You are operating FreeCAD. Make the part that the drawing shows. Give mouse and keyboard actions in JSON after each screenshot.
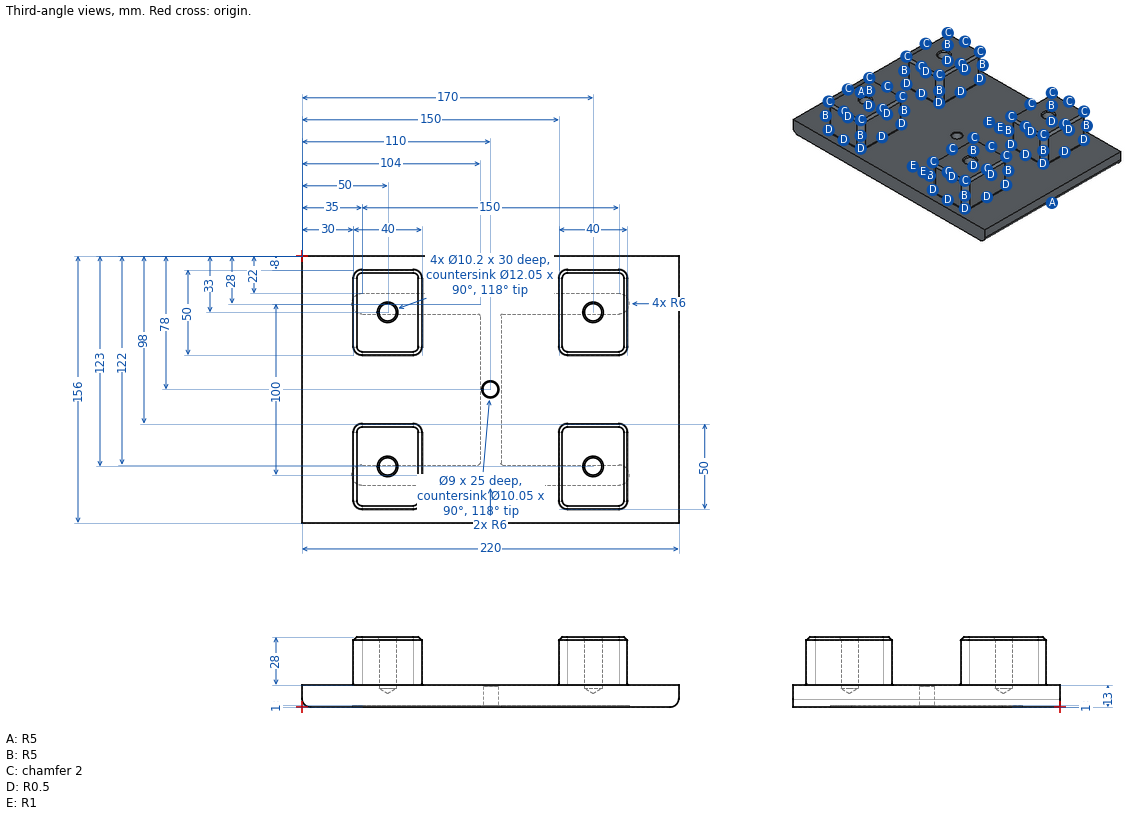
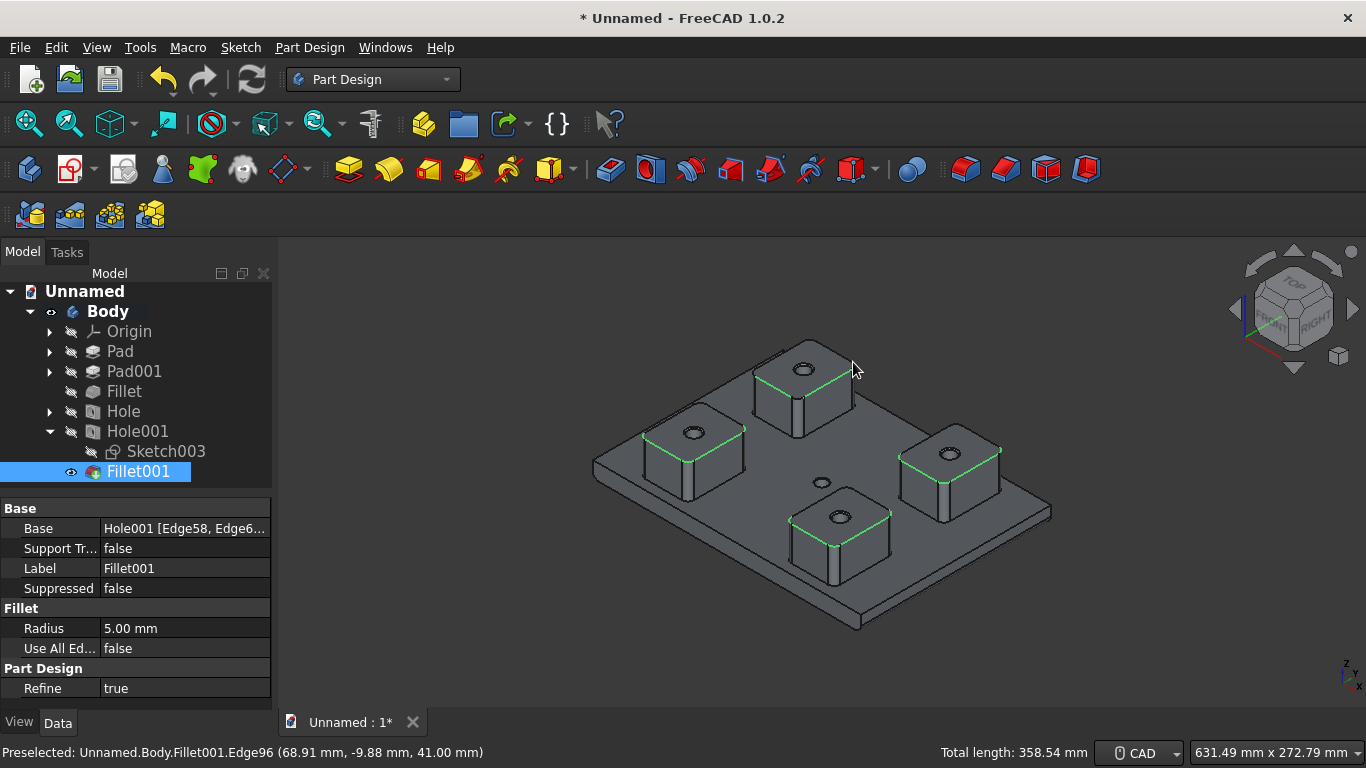
{"action": "left_click", "coordinate": [754, 369], "text": "ctrl"}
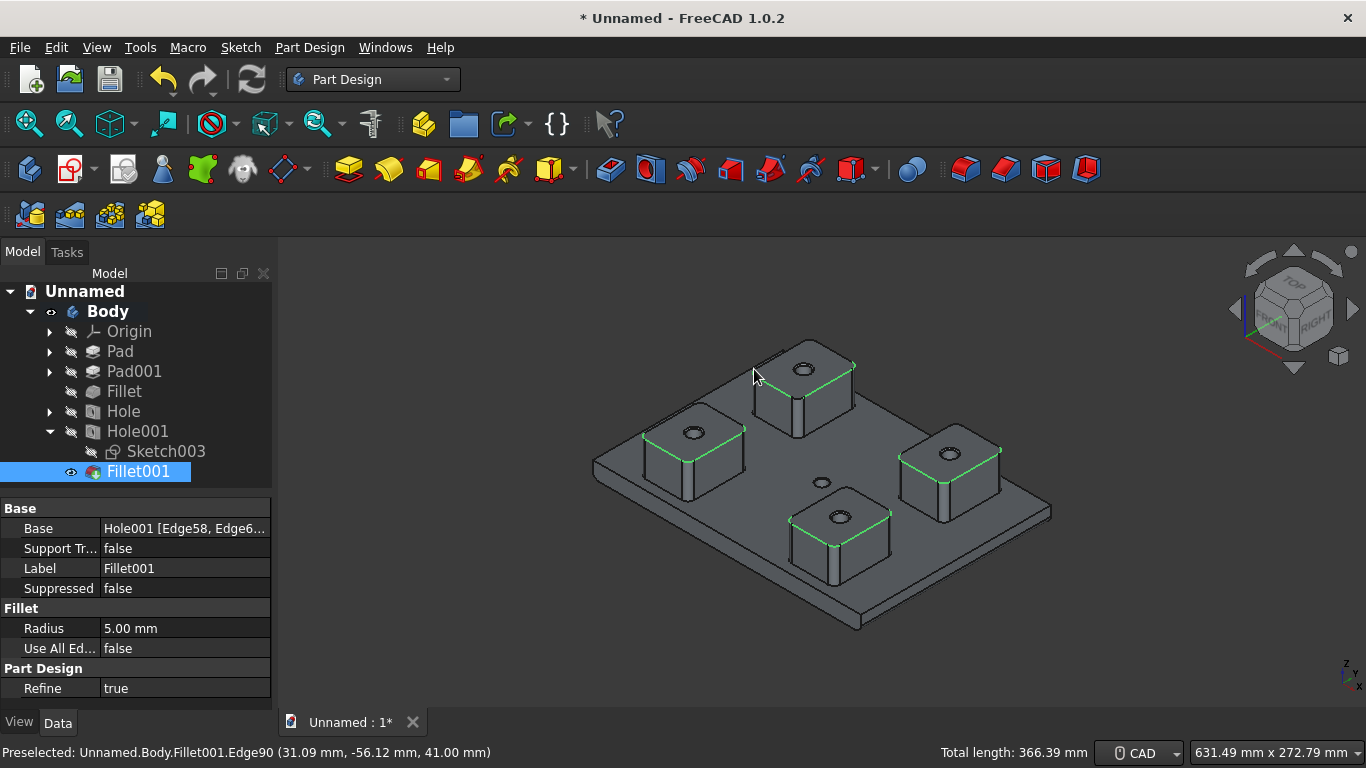
{"action": "left_click", "coordinate": [798, 398], "text": "ctrl"}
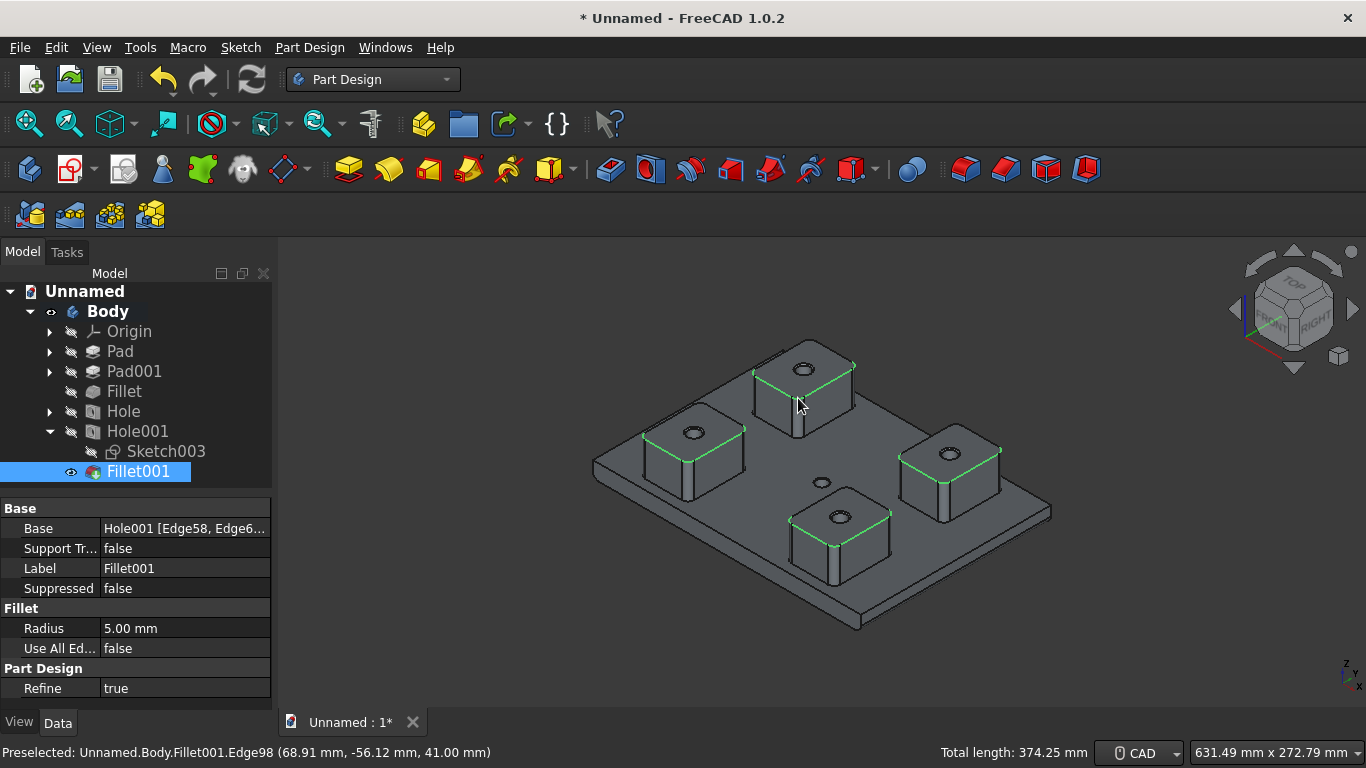
{"action": "key", "text": "2"}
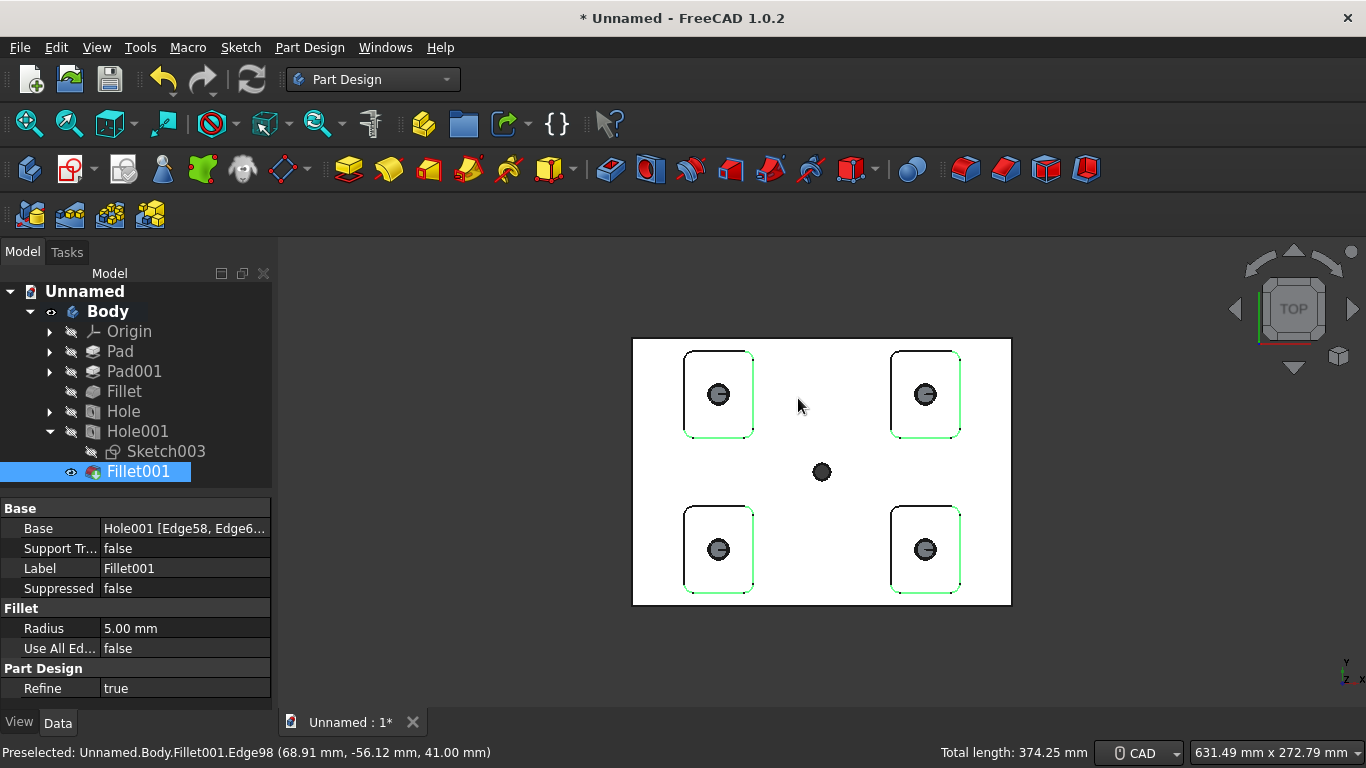
{"action": "left_click", "coordinate": [719, 505], "text": "ctrl"}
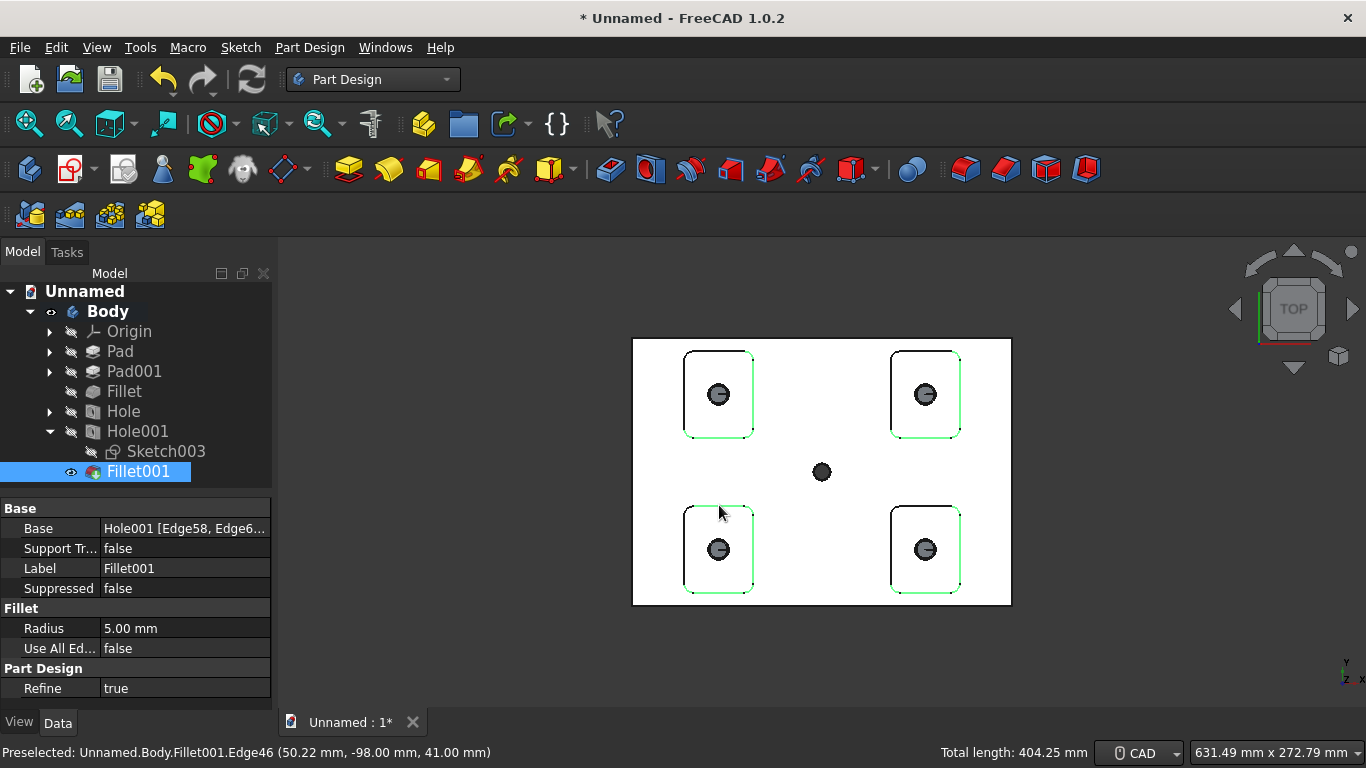
{"action": "left_click", "coordinate": [684, 549], "text": "ctrl"}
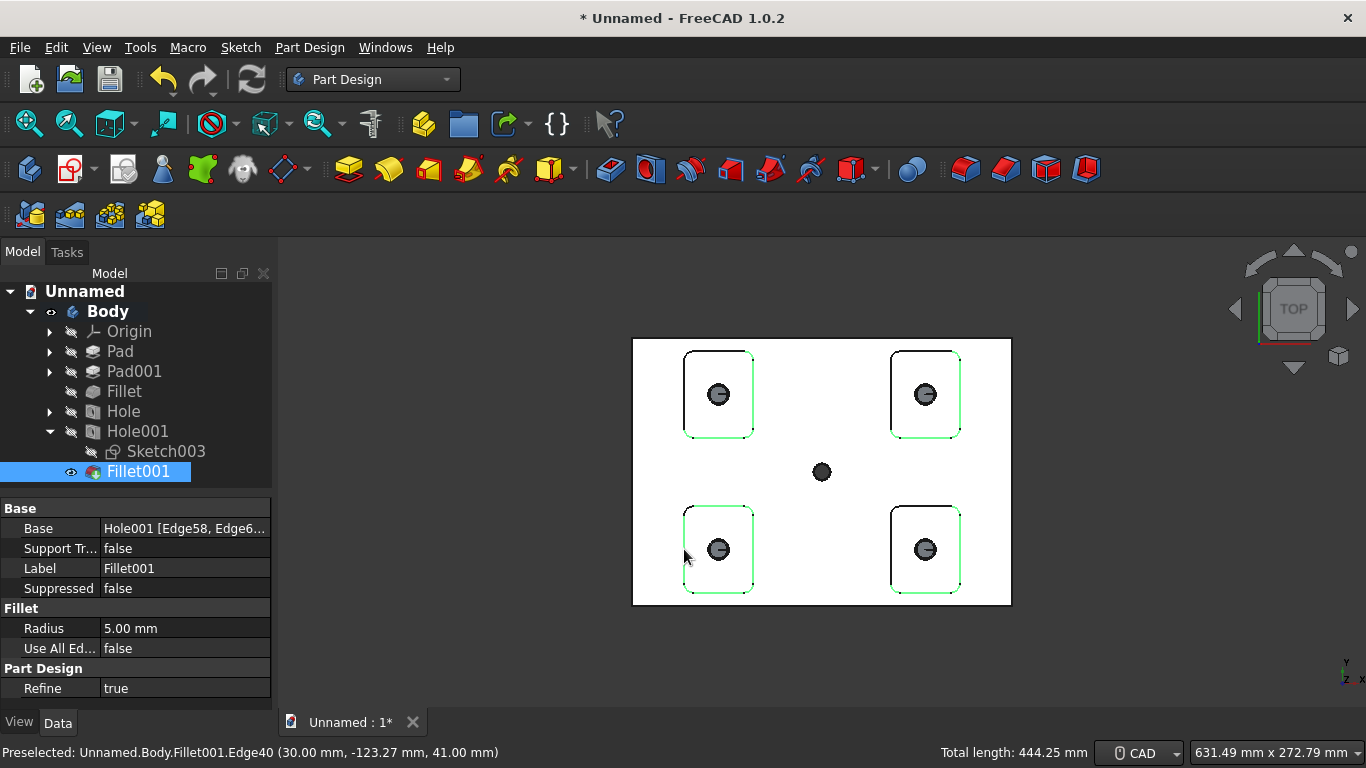
{"action": "left_click", "coordinate": [687, 508], "text": "ctrl"}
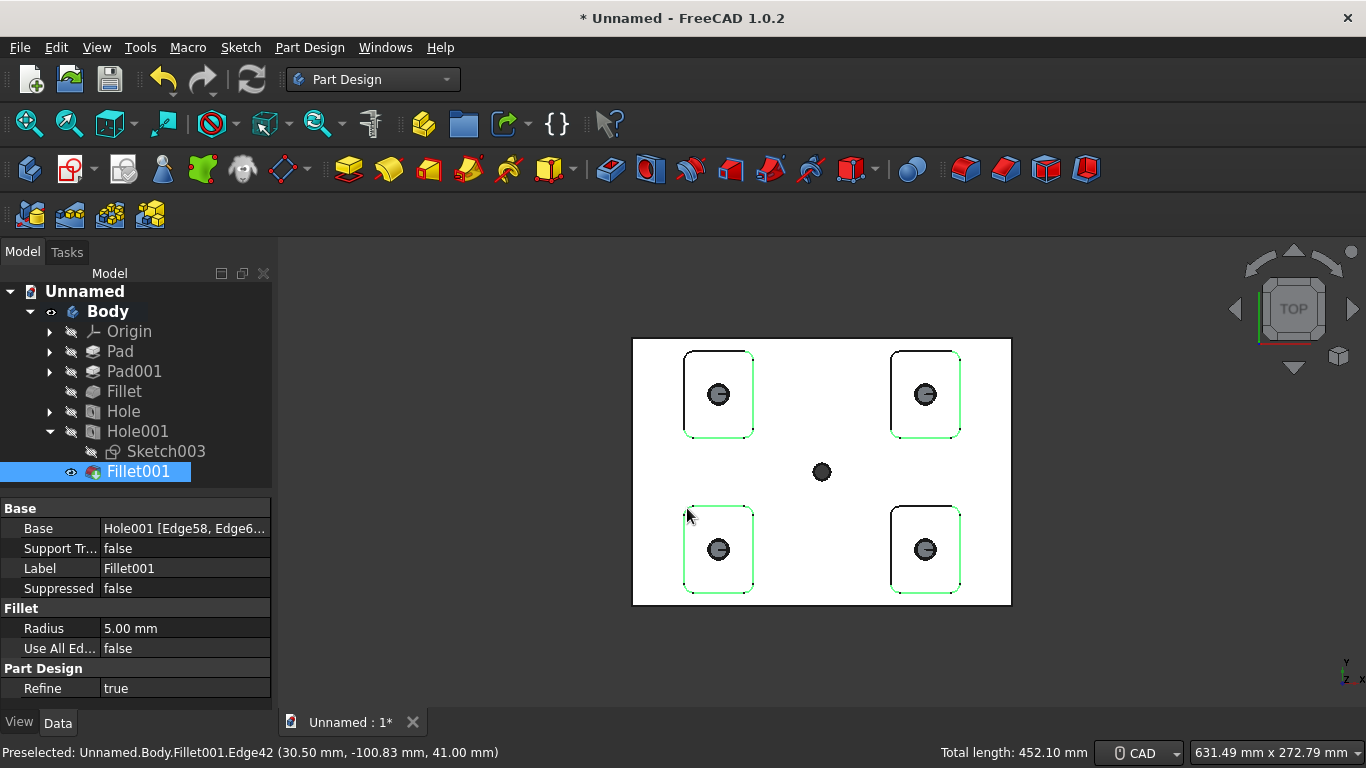
{"action": "left_click", "coordinate": [891, 549], "text": "ctrl"}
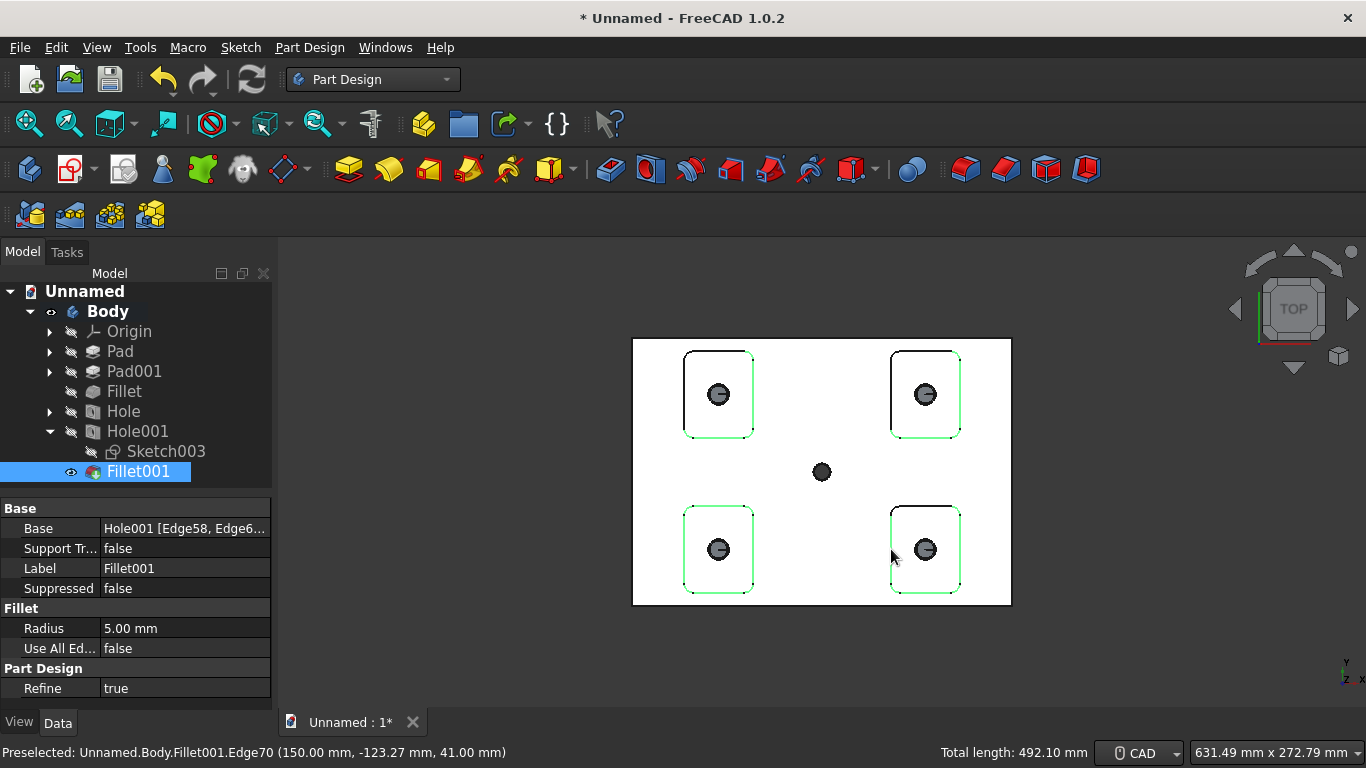
{"action": "left_click", "coordinate": [925, 505], "text": "ctrl"}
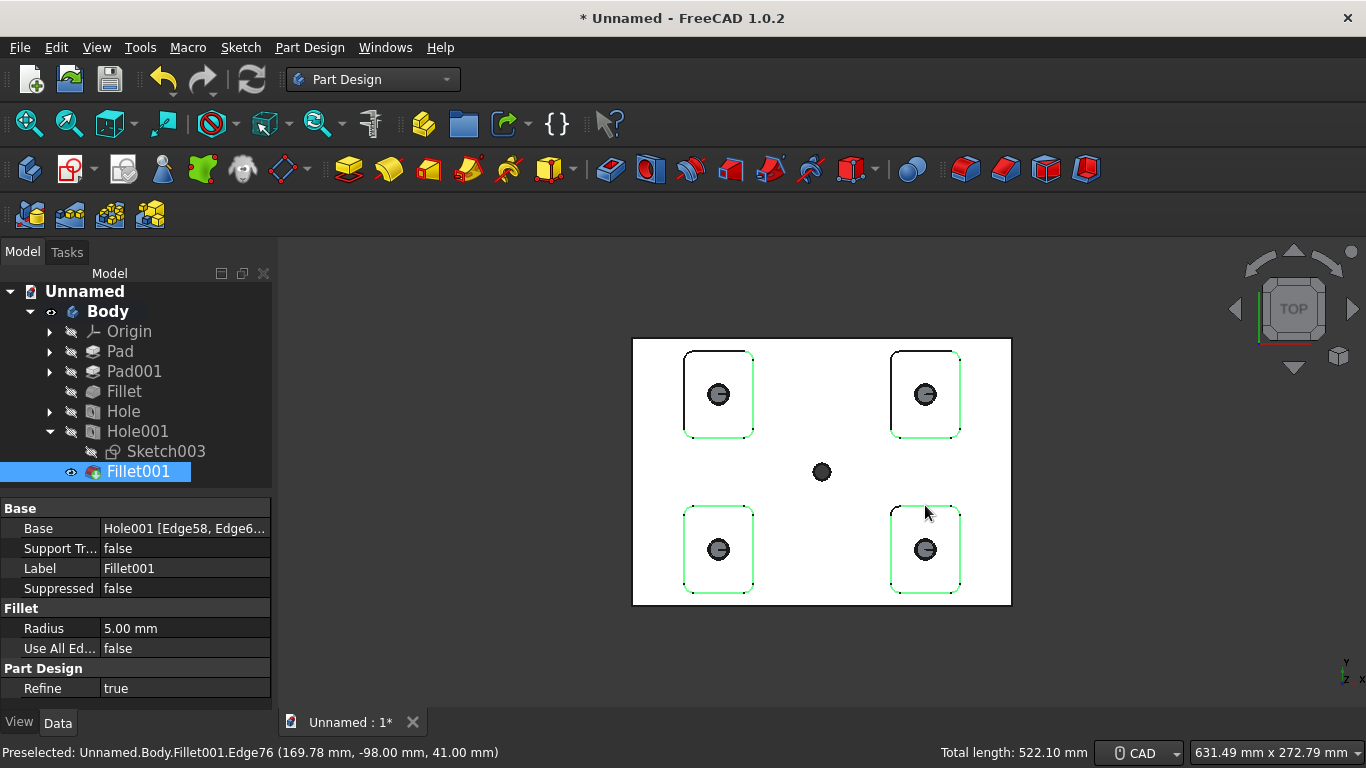
{"action": "left_click", "coordinate": [893, 508], "text": "ctrl"}